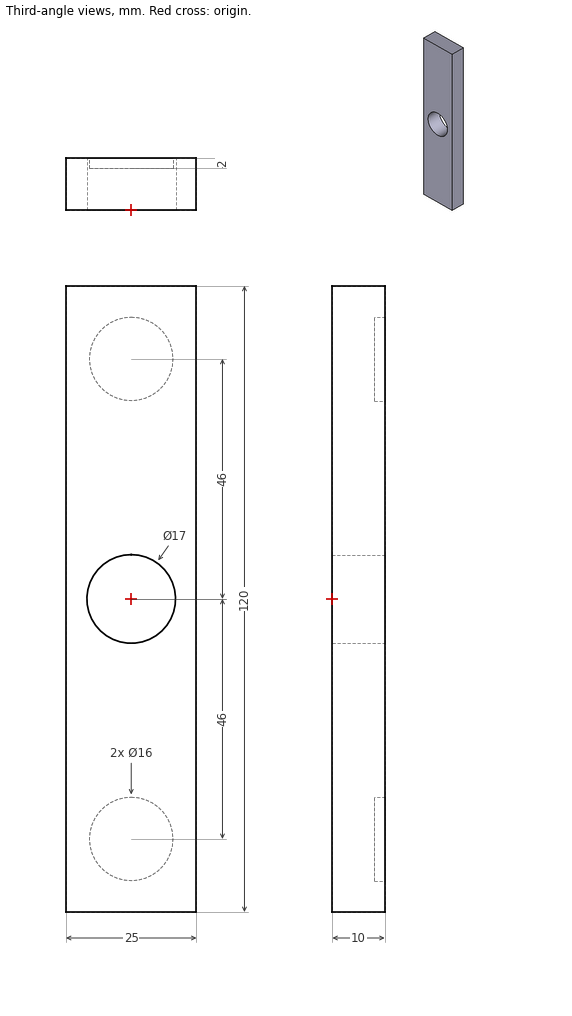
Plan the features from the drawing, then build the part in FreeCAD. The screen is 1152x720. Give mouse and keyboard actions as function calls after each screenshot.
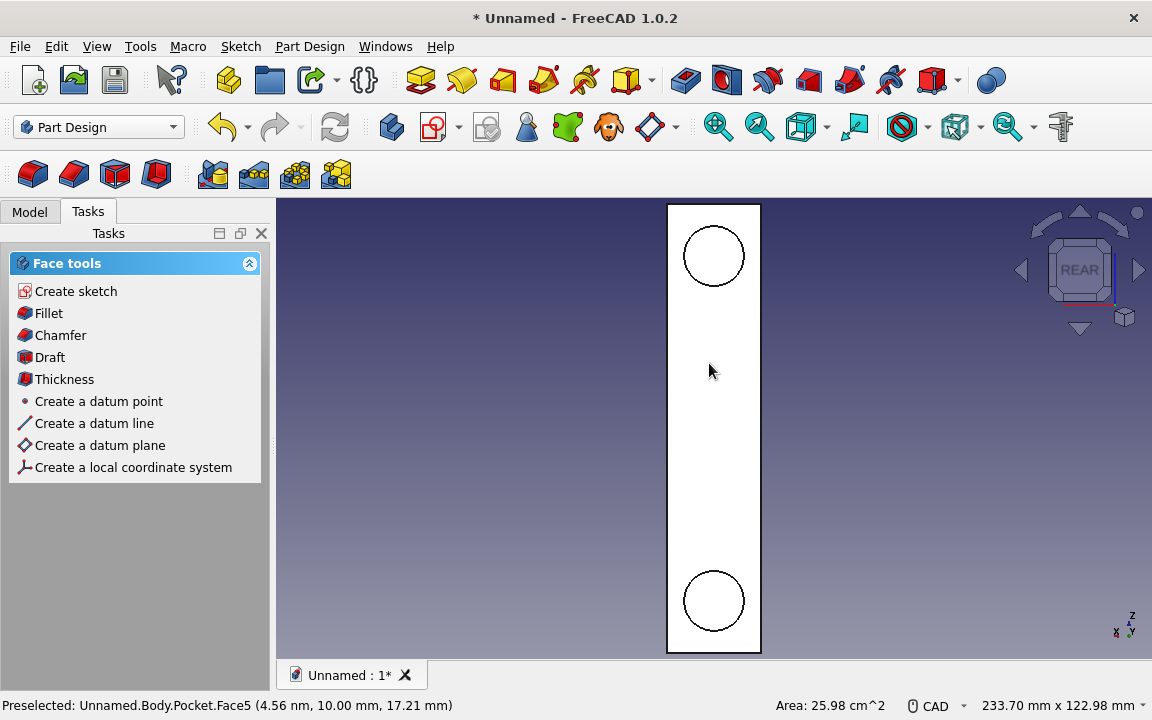
click(432, 128)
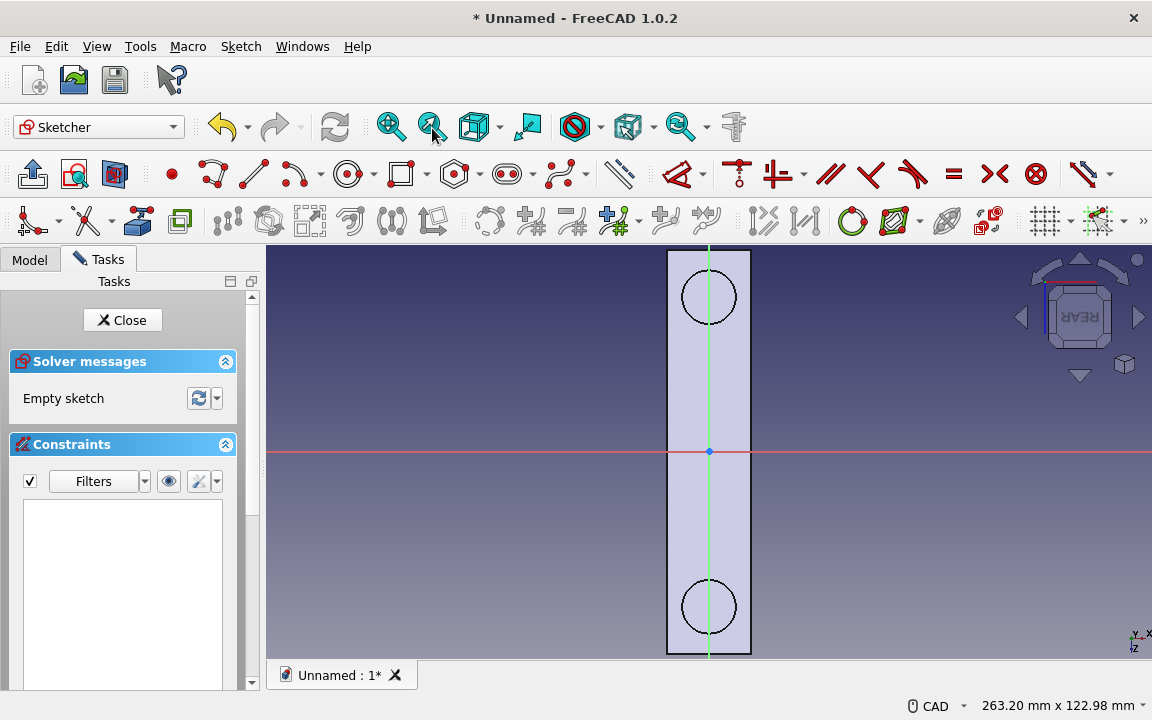
scroll(731, 452, up, 7)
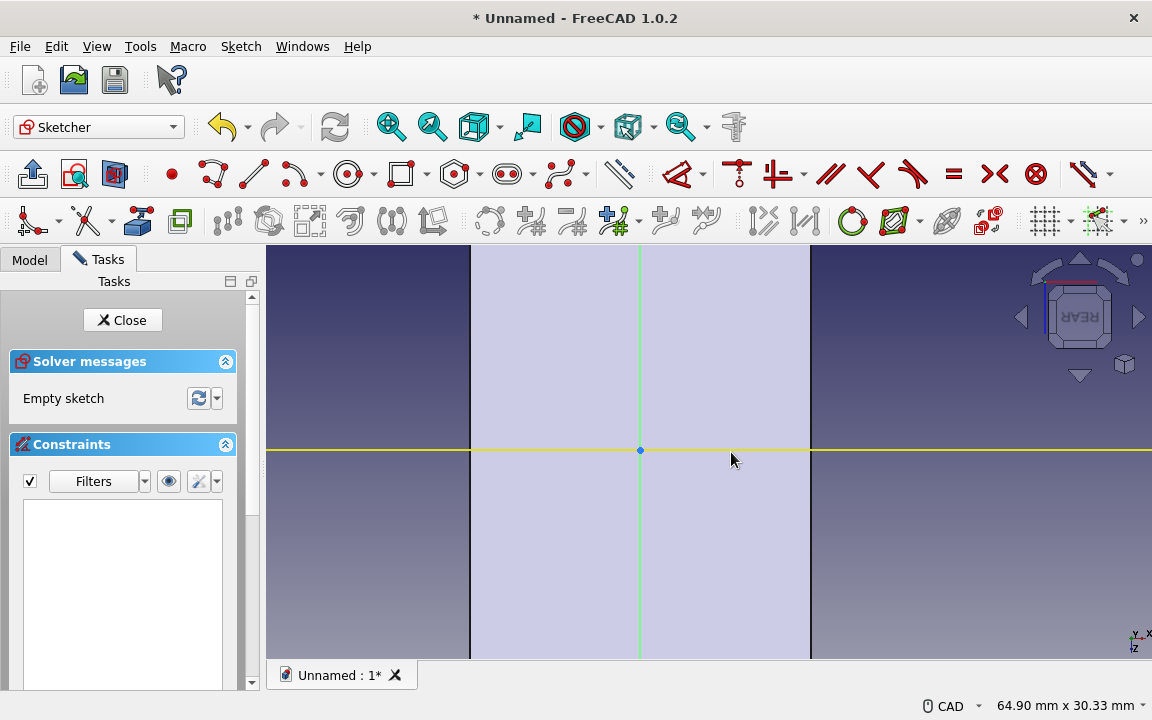
click(348, 174)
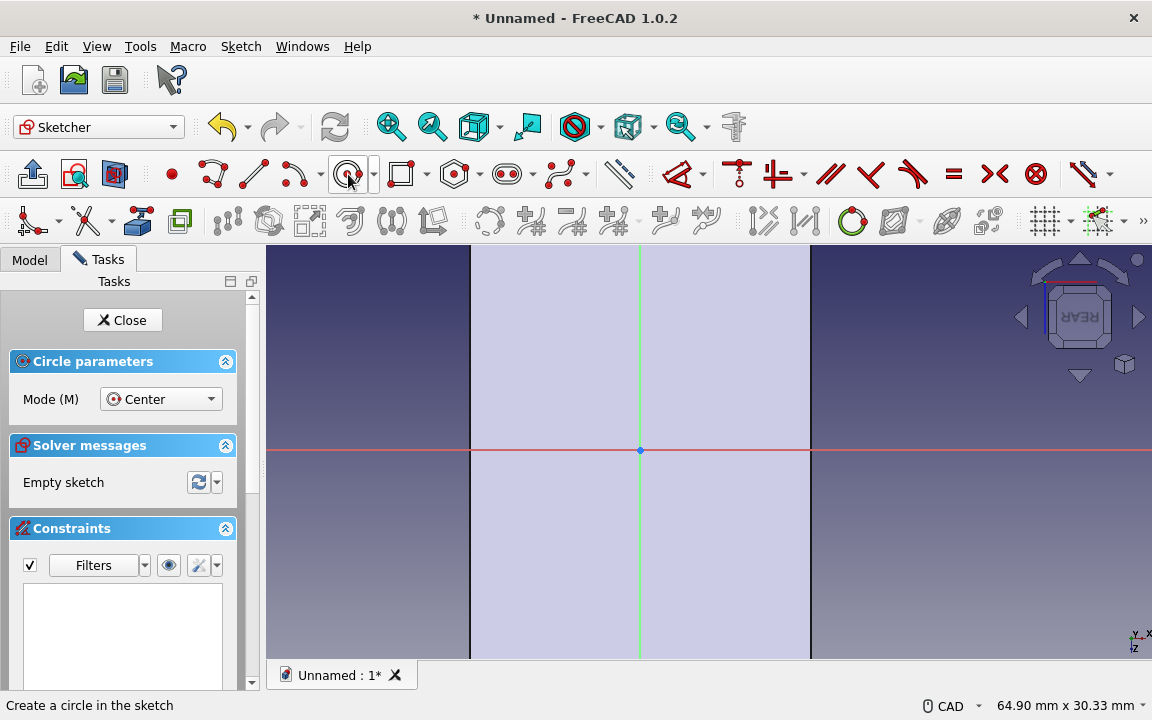
click(640, 450)
move(722, 368)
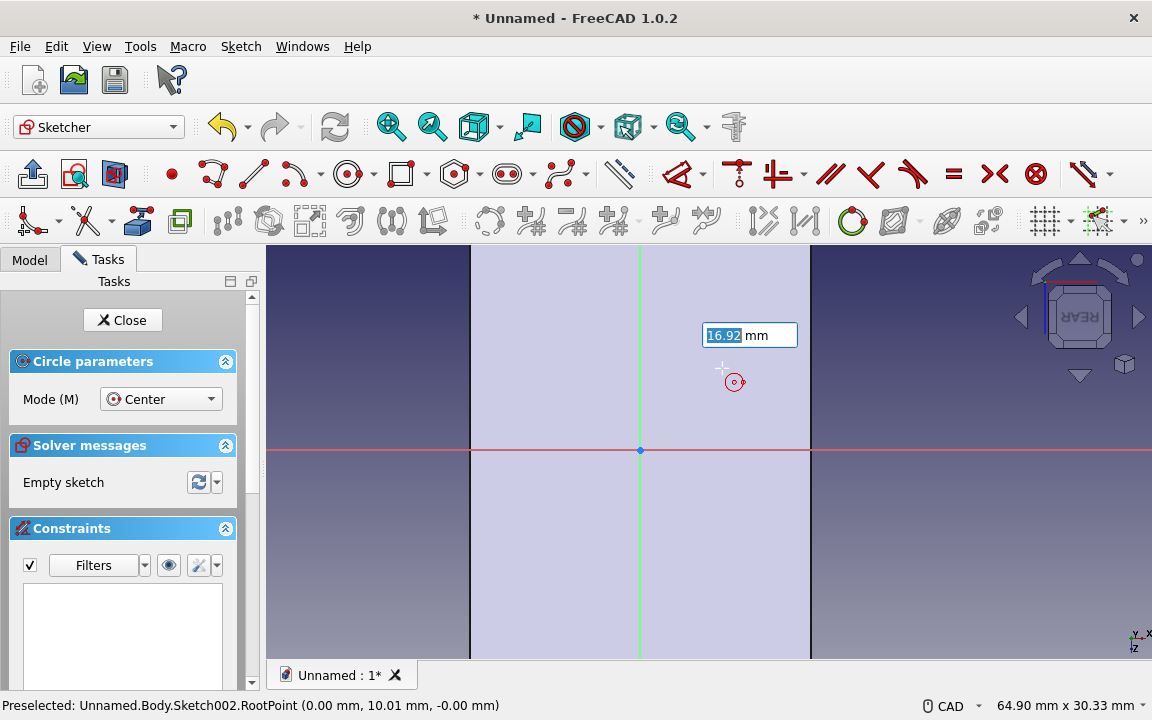
text(17)
key(Return)
key(Escape)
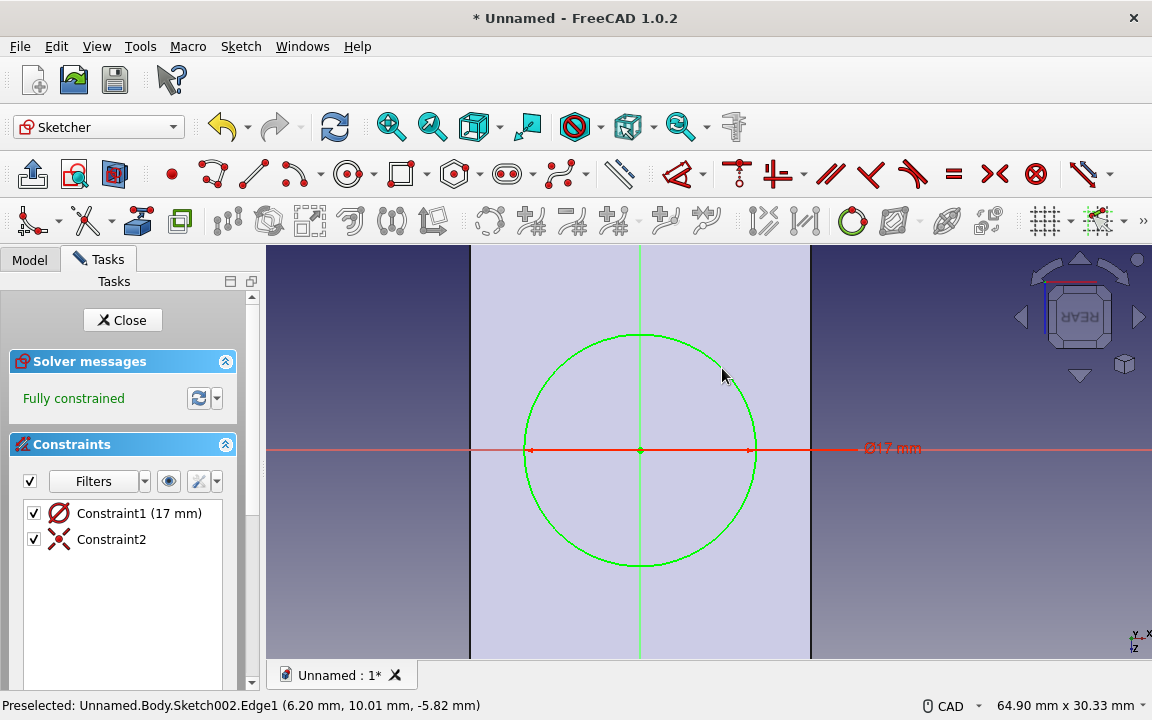
click(123, 320)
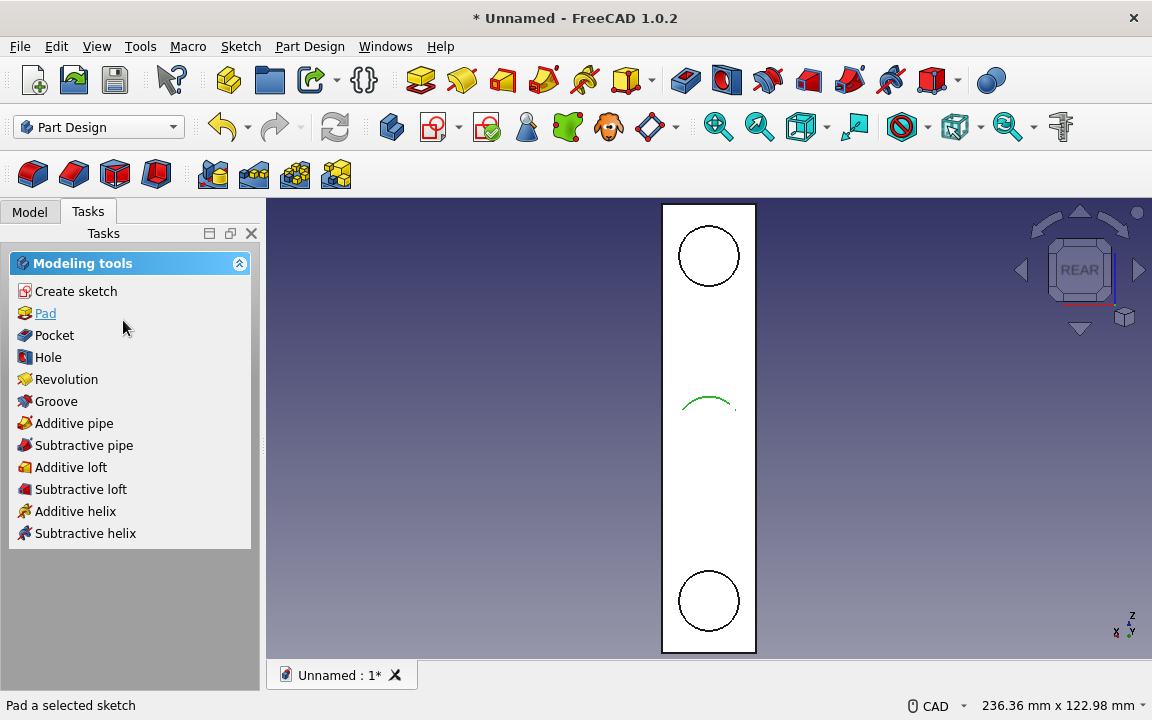
click(686, 80)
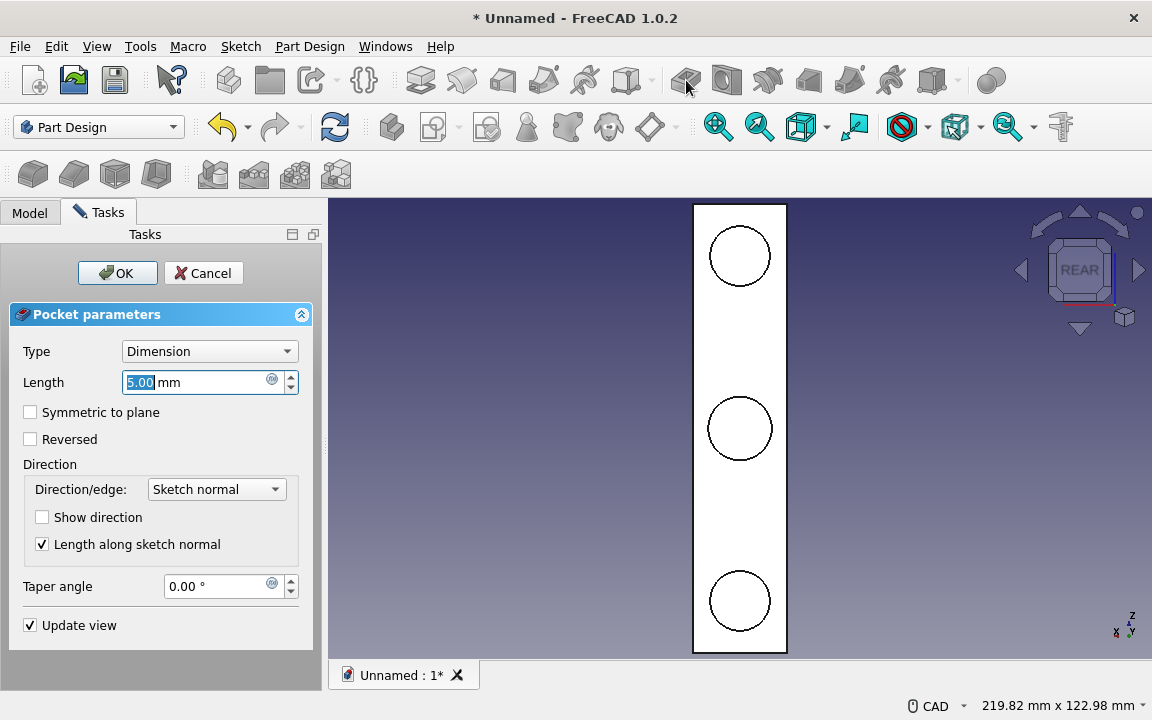
click(210, 352)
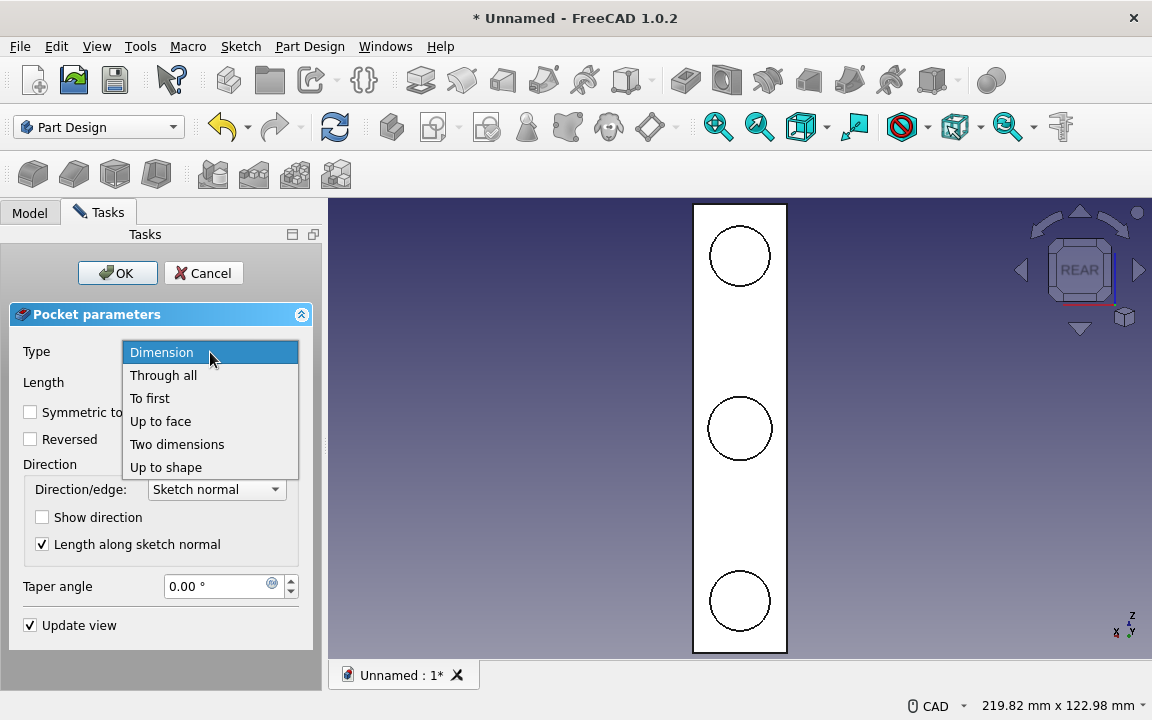
click(208, 398)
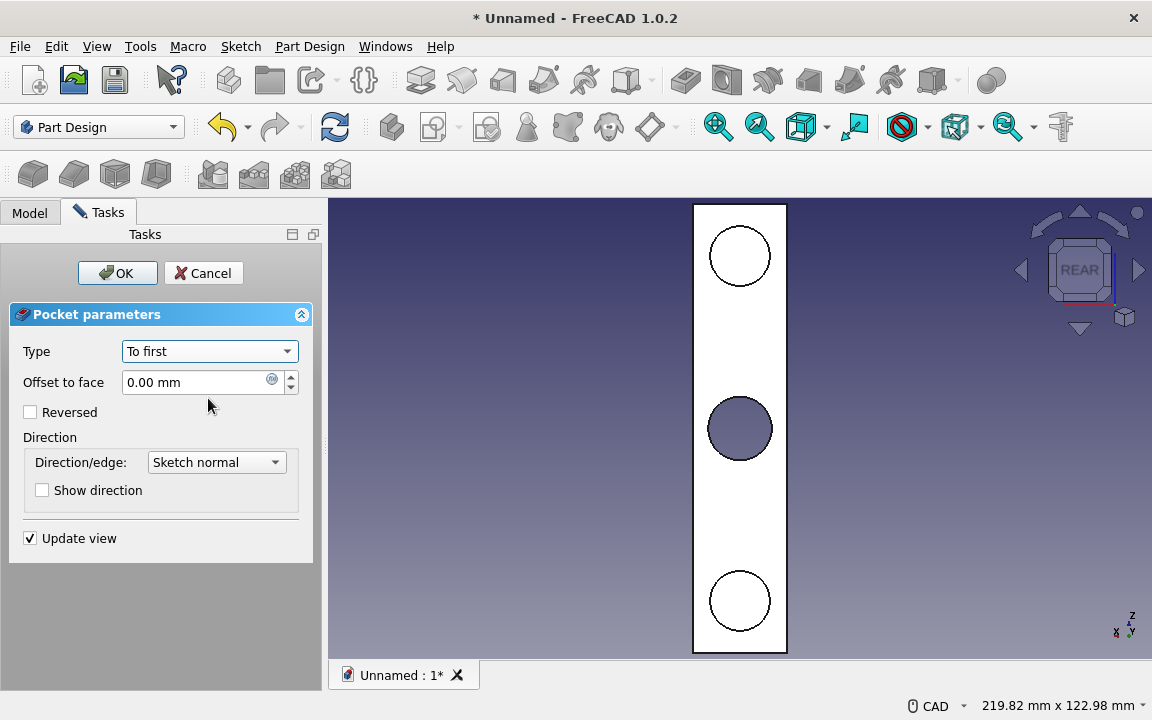
click(118, 273)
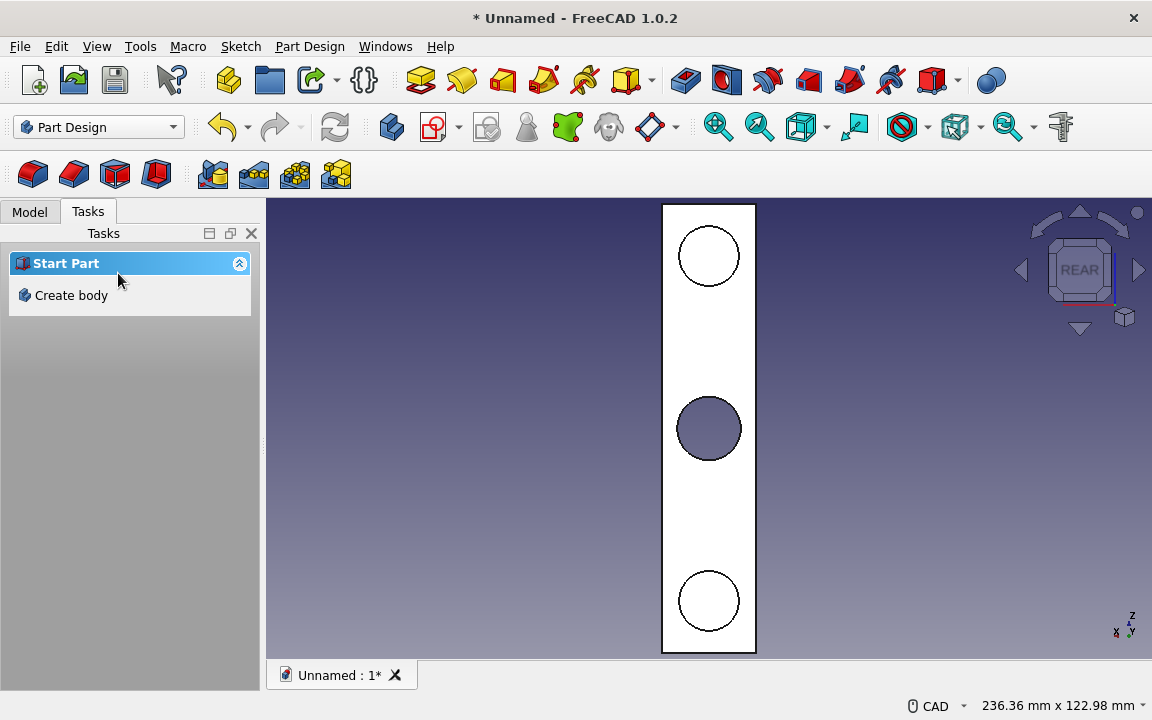
key(0)